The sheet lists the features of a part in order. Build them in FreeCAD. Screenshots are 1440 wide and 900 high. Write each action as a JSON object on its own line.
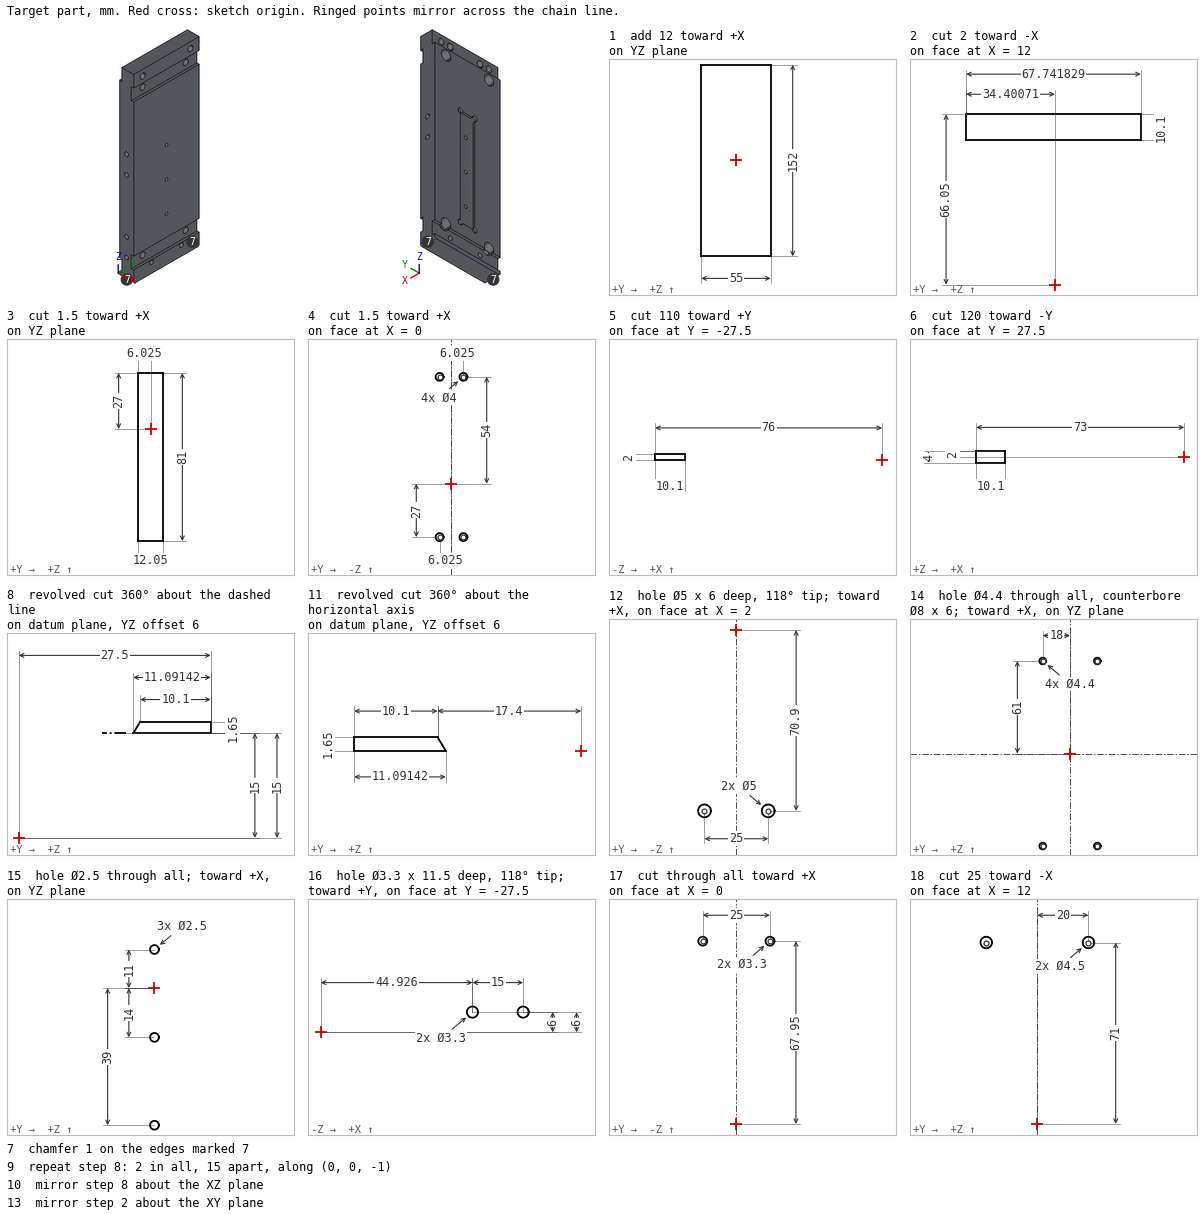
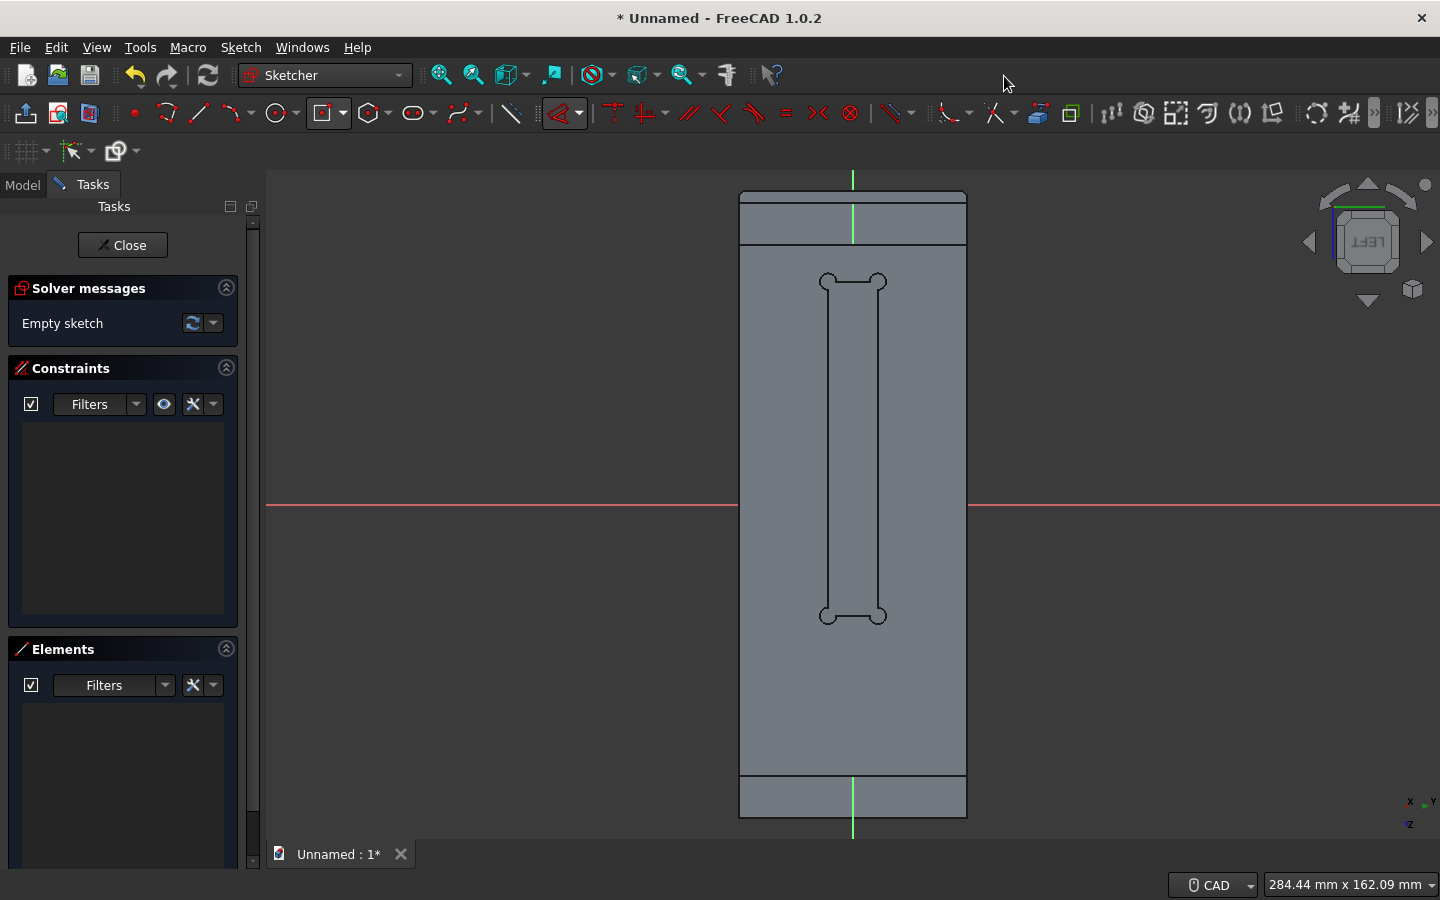
{"action": "scroll", "coordinate": [475, 198], "scroll_direction": "down", "scroll_amount": 1}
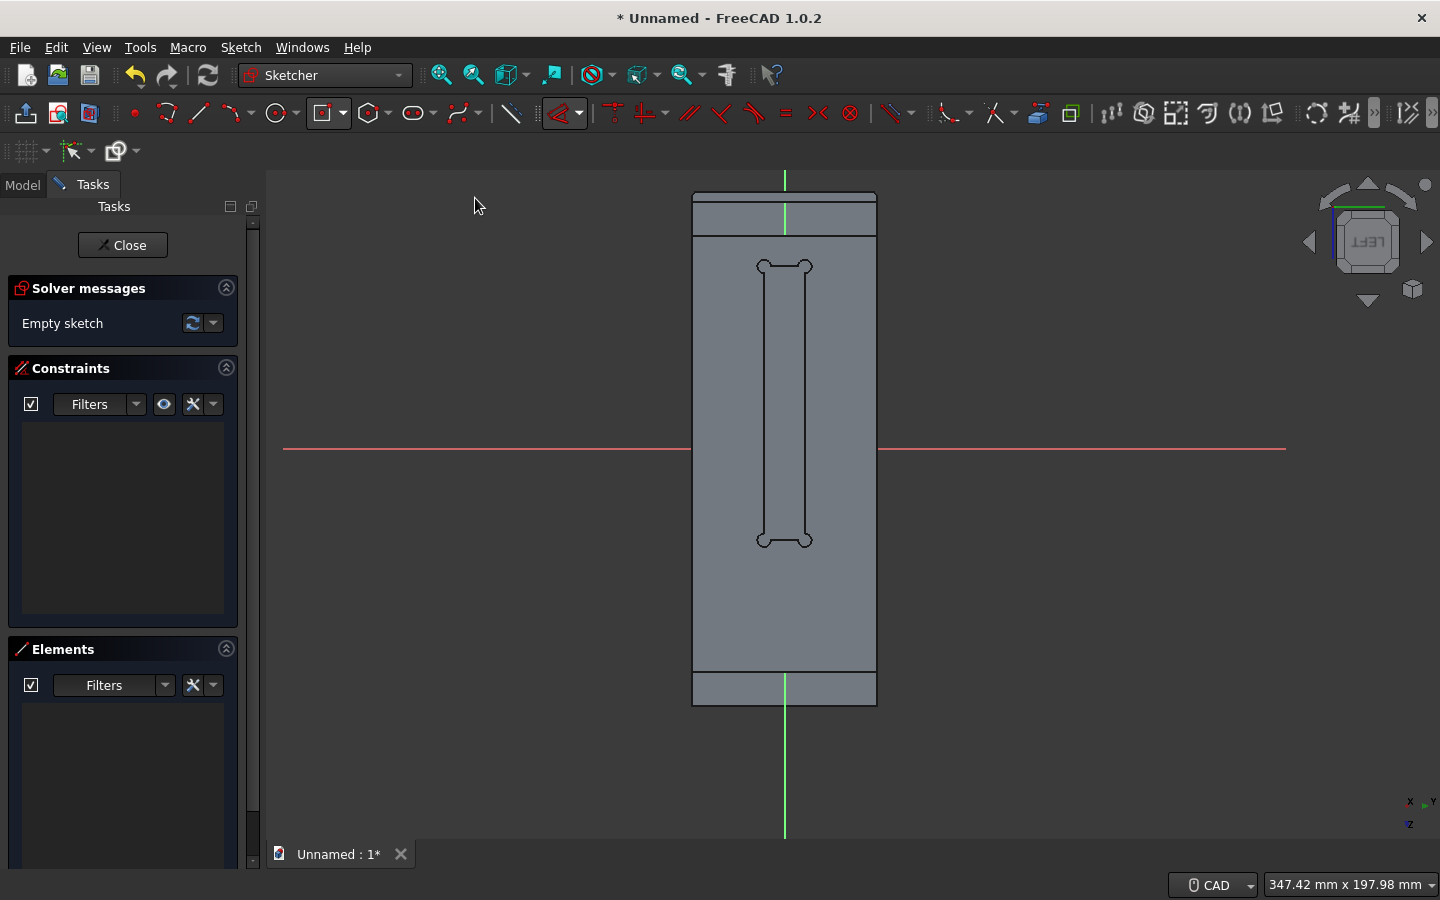
{"action": "scroll", "coordinate": [785, 656], "scroll_direction": "up", "scroll_amount": 3}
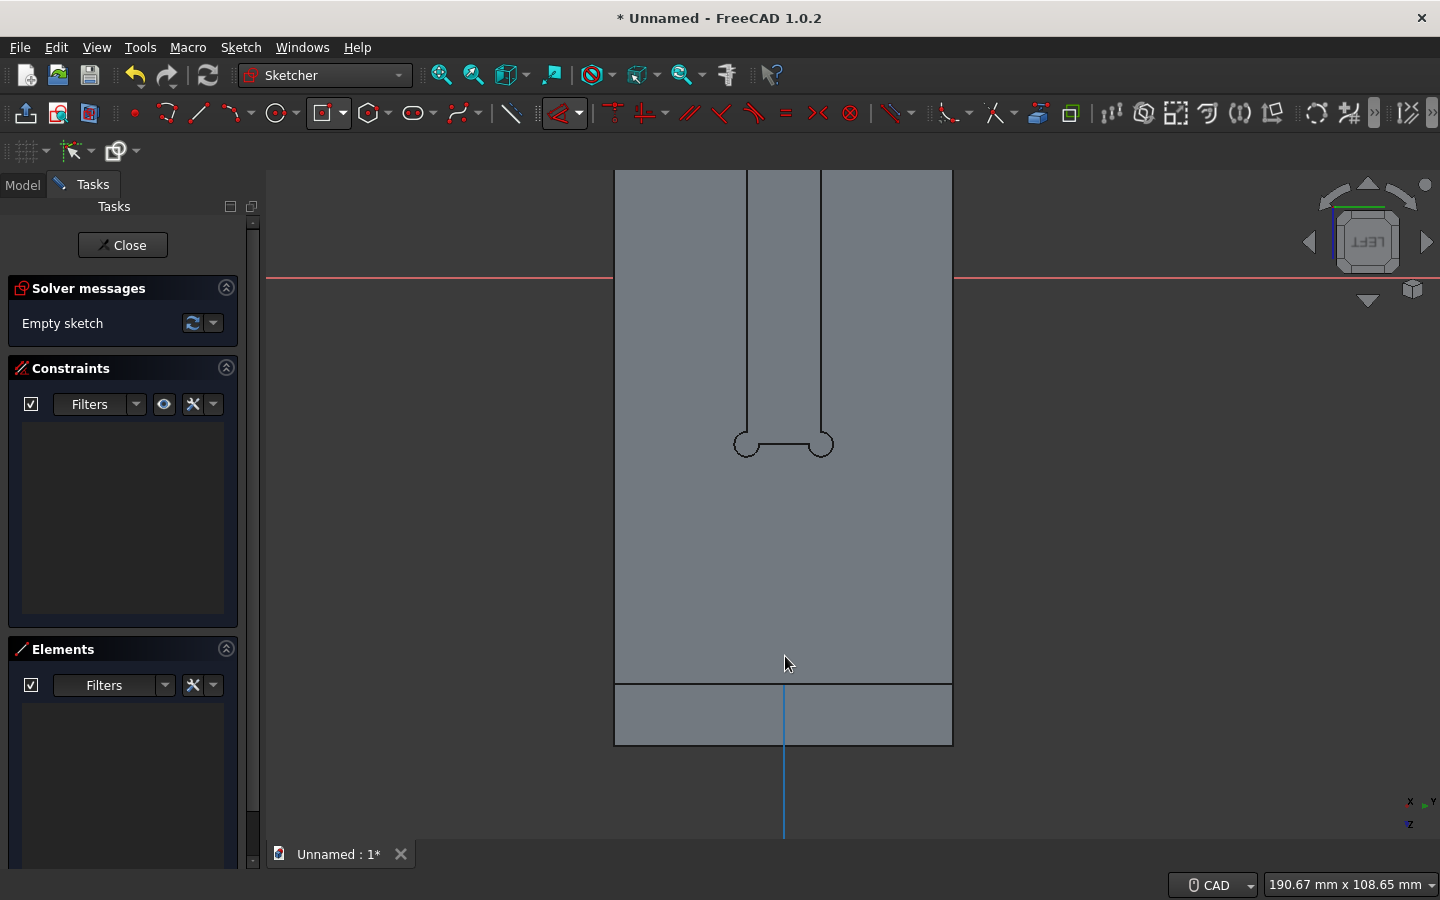
{"action": "left_click", "coordinate": [276, 114]}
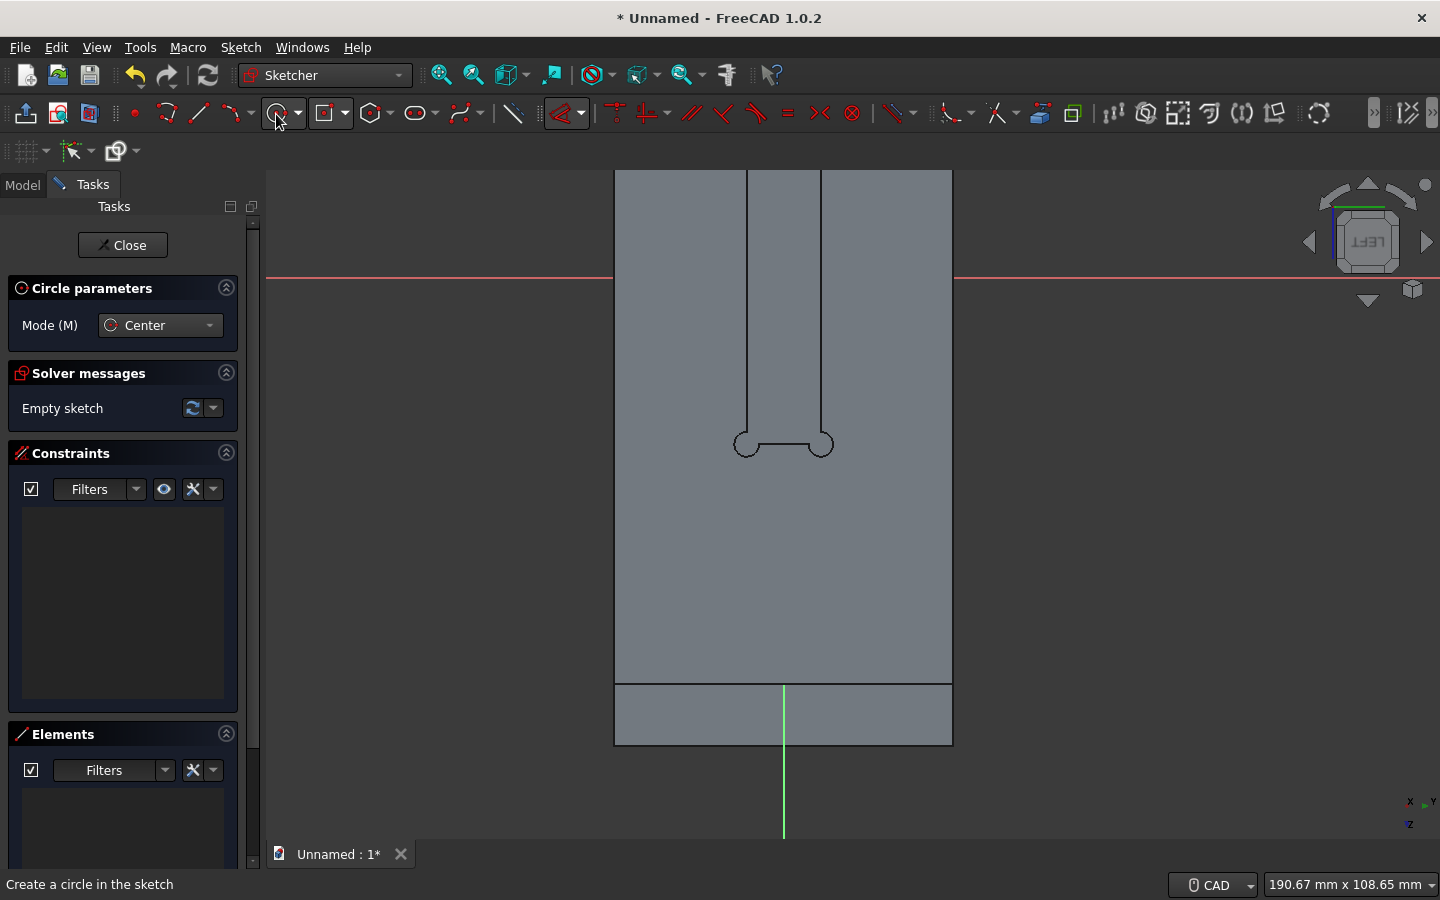
{"action": "scroll", "coordinate": [861, 715], "scroll_direction": "up", "scroll_amount": 2}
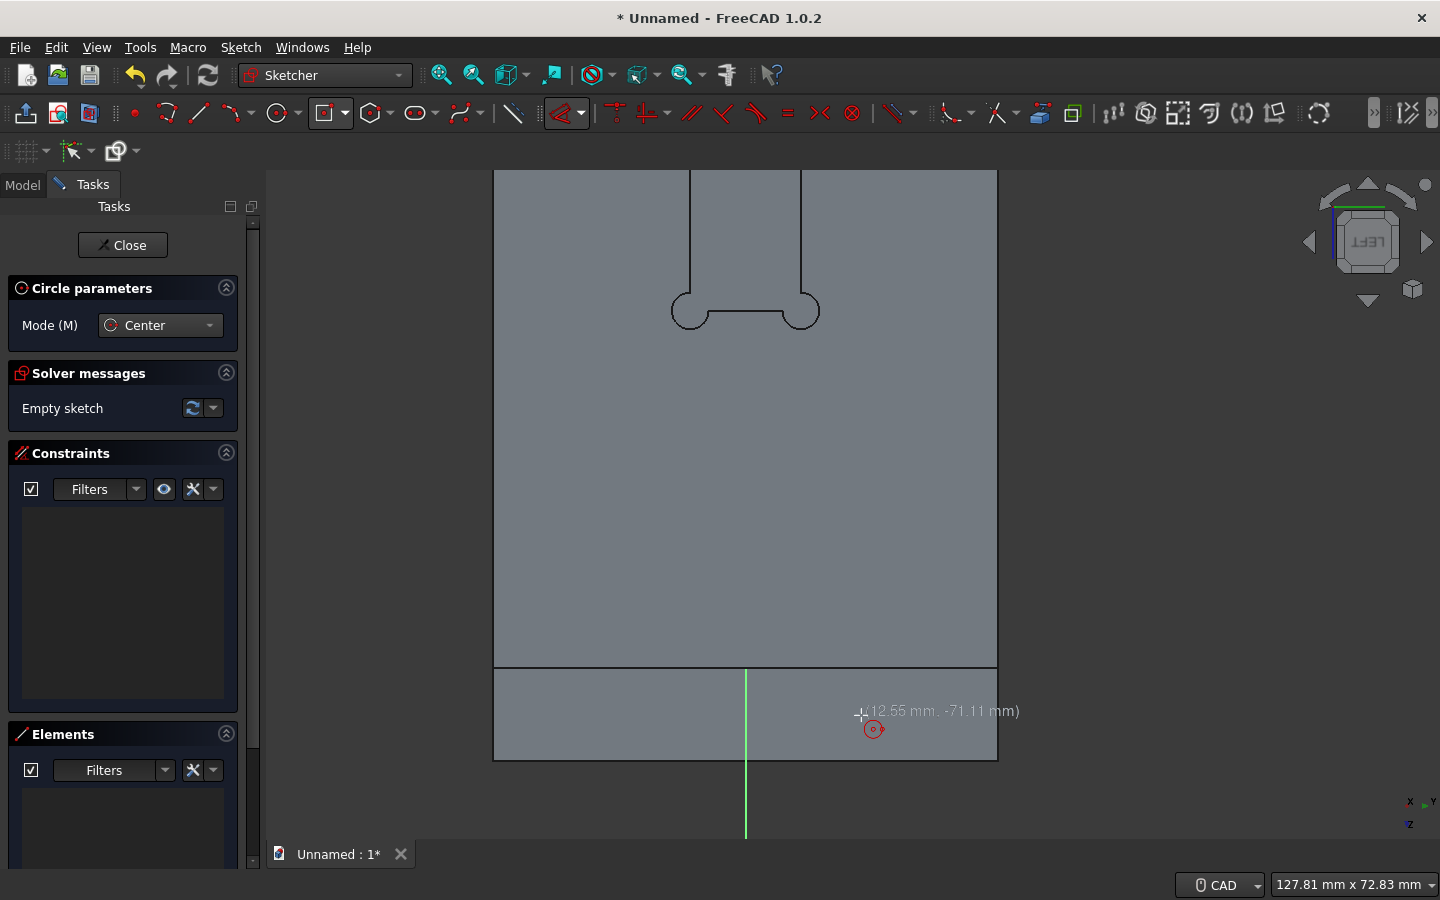
{"action": "left_click", "coordinate": [860, 714]}
{"action": "mouse_move", "coordinate": [877, 698]}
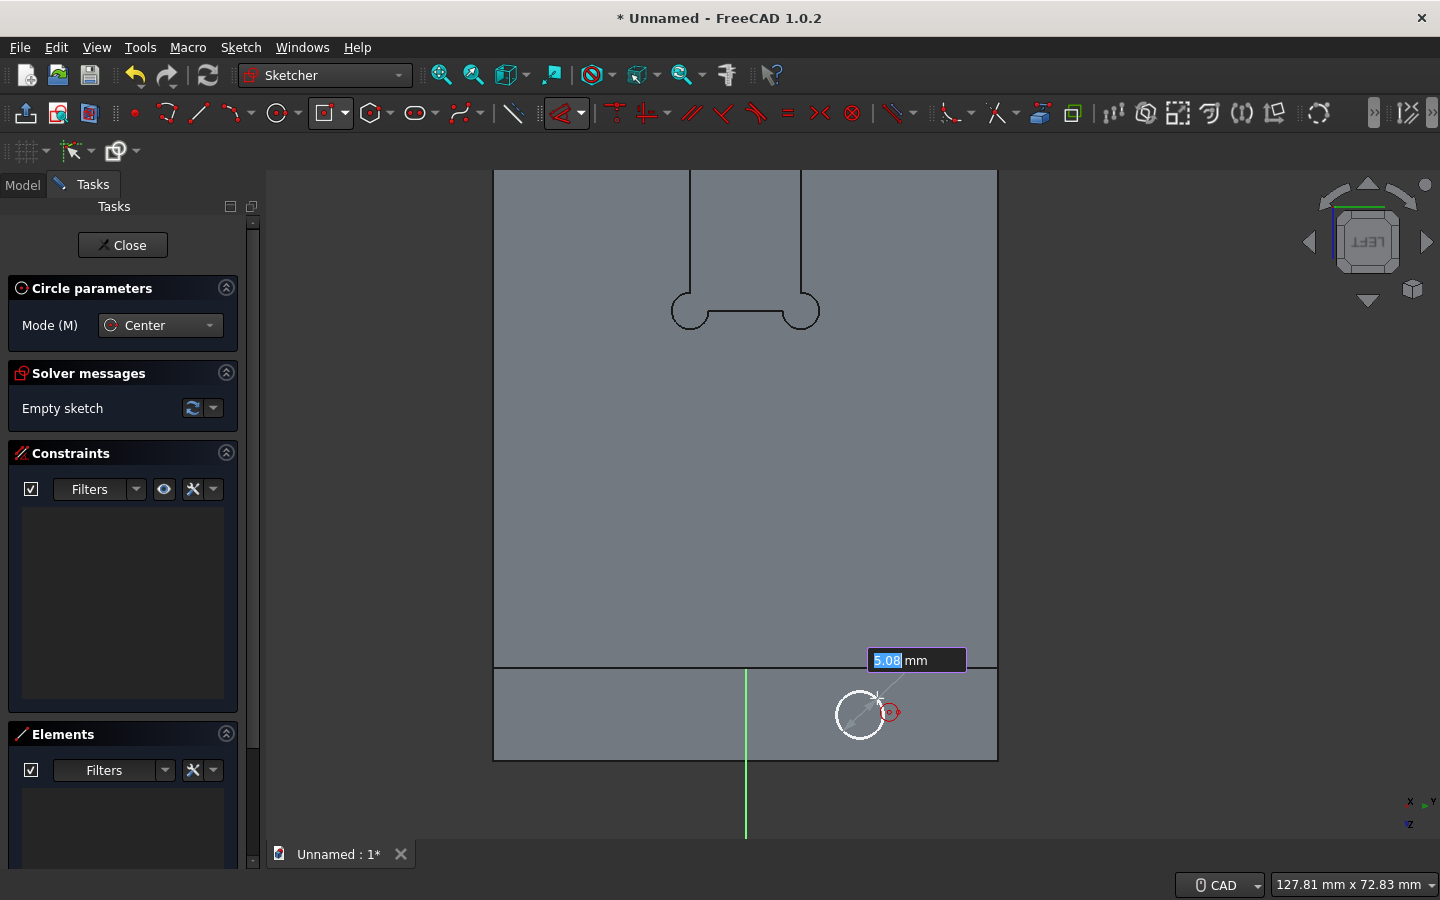
{"action": "type", "text": "5"}
{"action": "key", "text": "Return"}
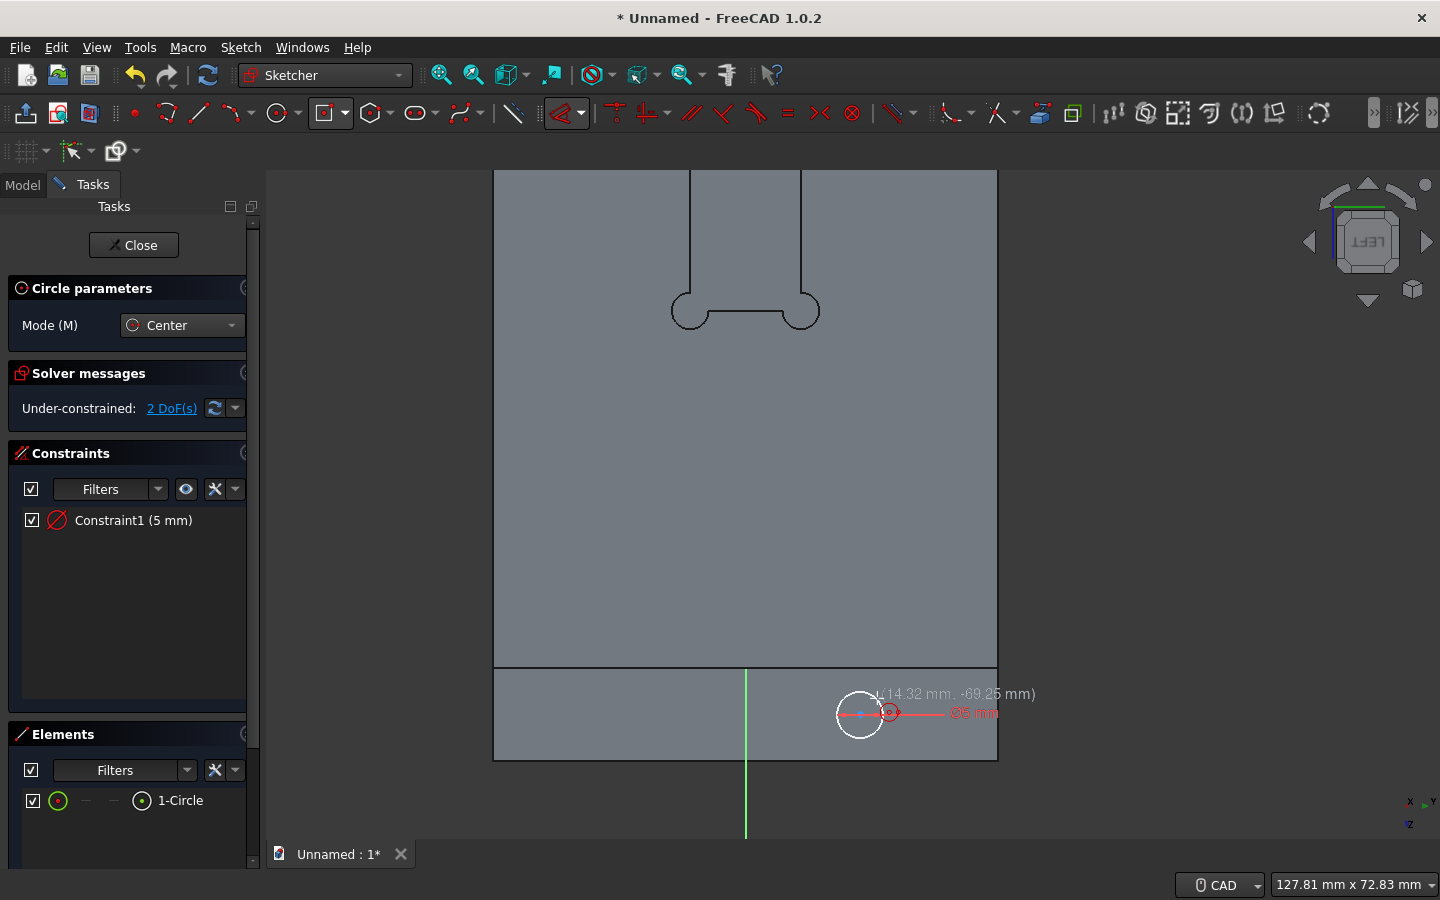
{"action": "left_click", "coordinate": [631, 714]}
{"action": "mouse_move", "coordinate": [647, 698]}